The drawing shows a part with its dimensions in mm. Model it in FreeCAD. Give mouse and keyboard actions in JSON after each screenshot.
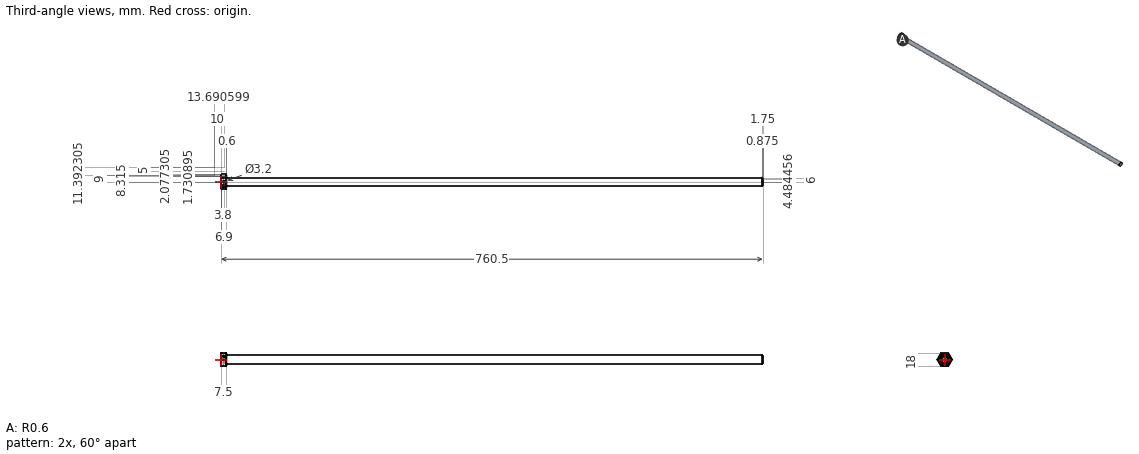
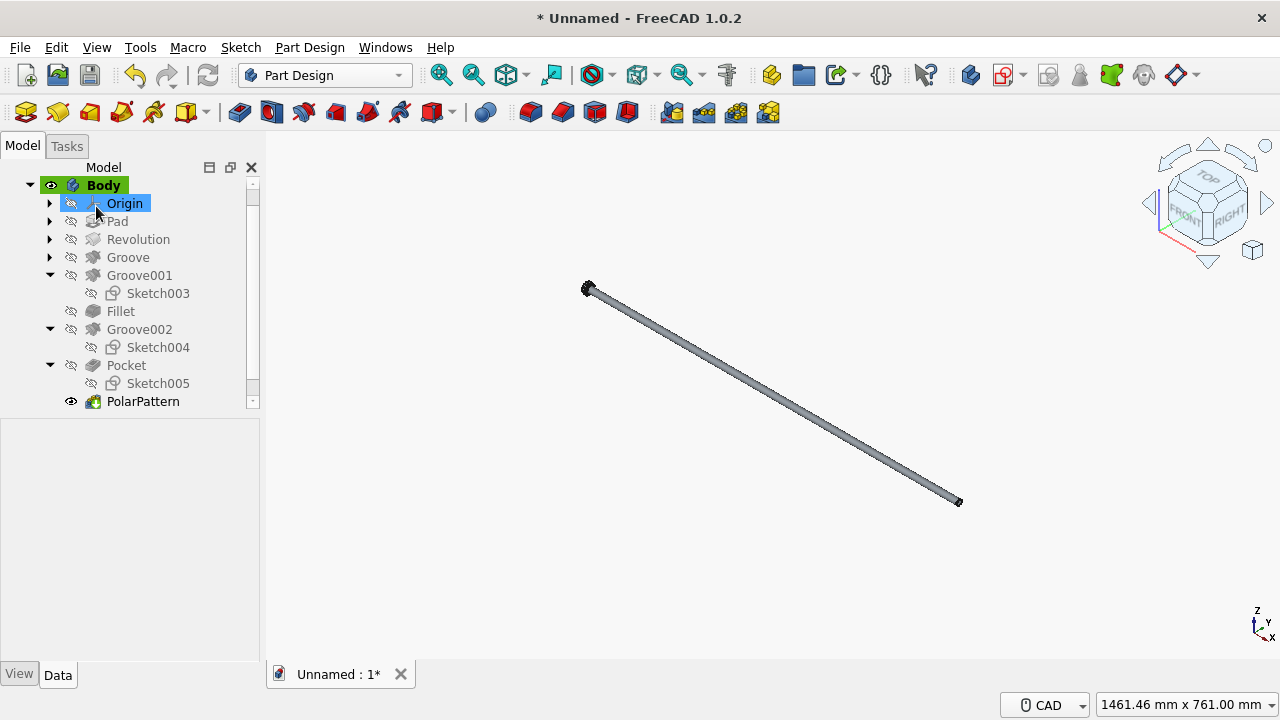
{"action": "key", "text": "v f"}